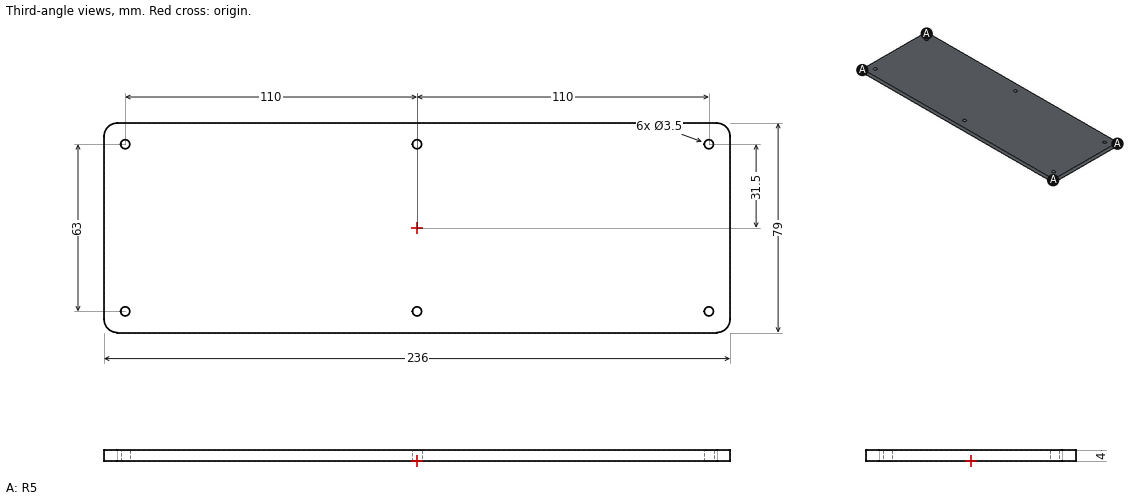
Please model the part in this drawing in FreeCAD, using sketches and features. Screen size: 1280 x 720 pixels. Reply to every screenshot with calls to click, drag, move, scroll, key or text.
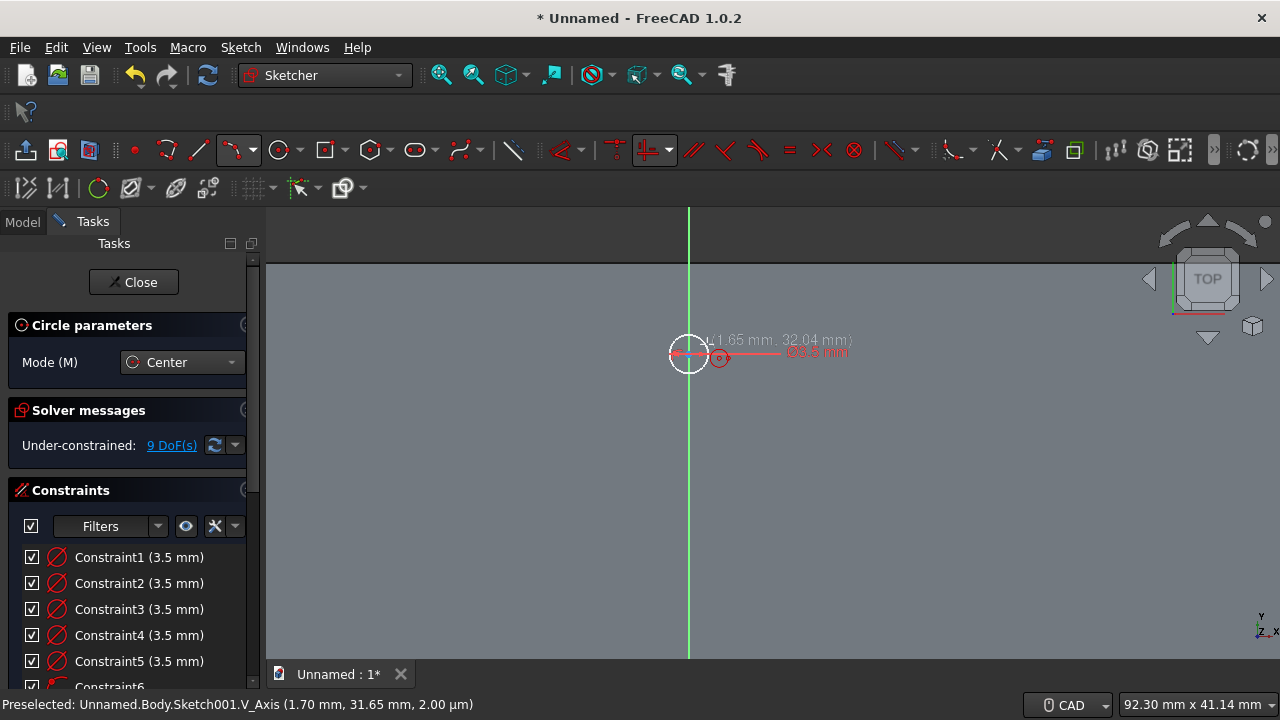
scroll(710, 347, down, 7)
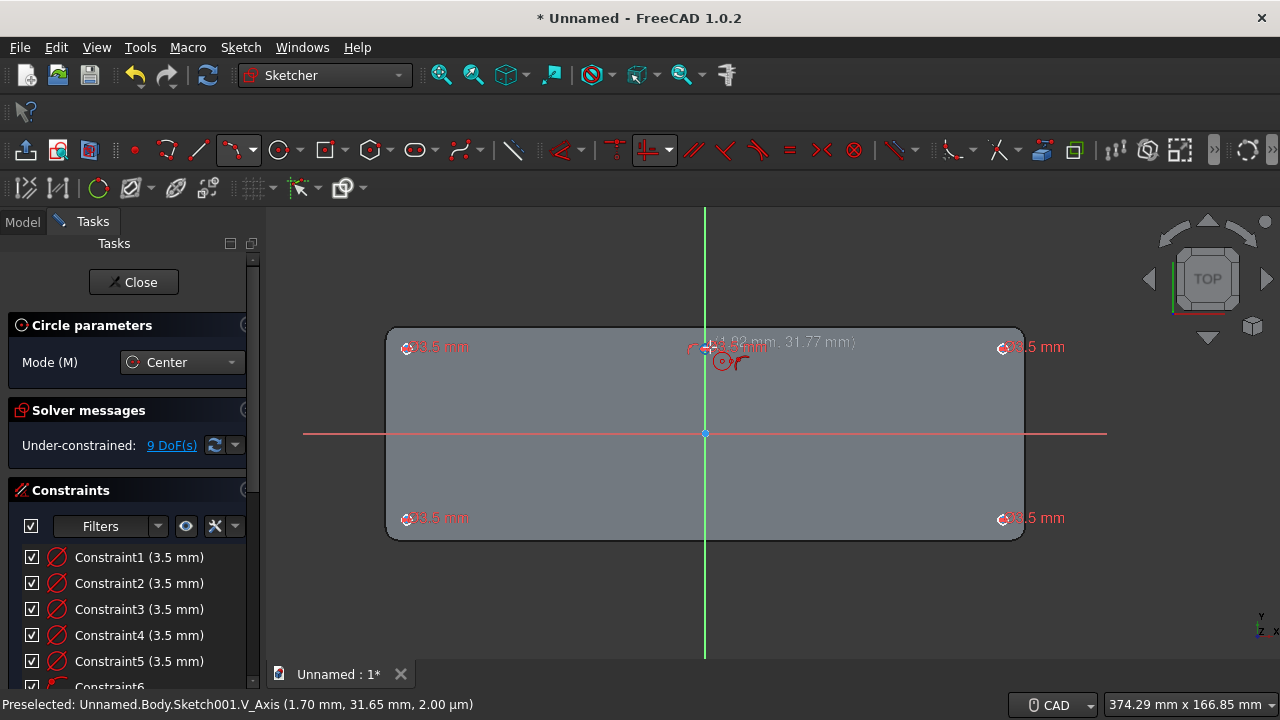
scroll(705, 519, up, 8)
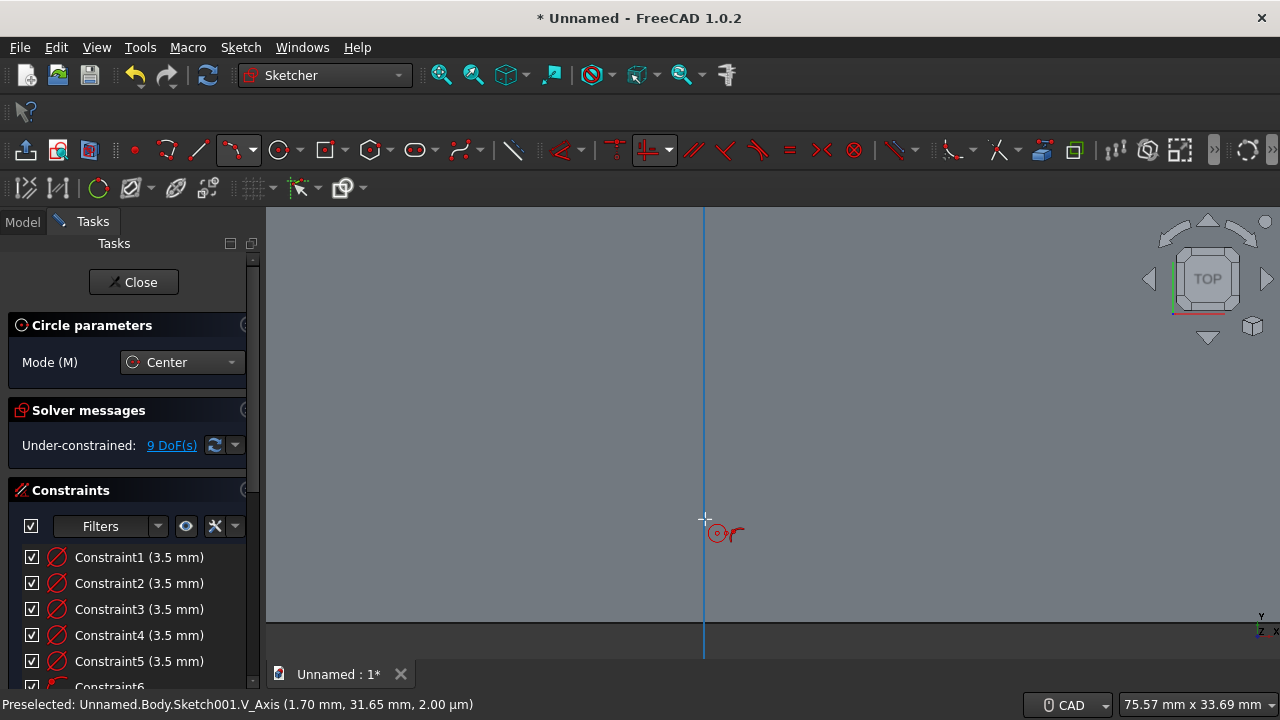
scroll(705, 519, down, 8)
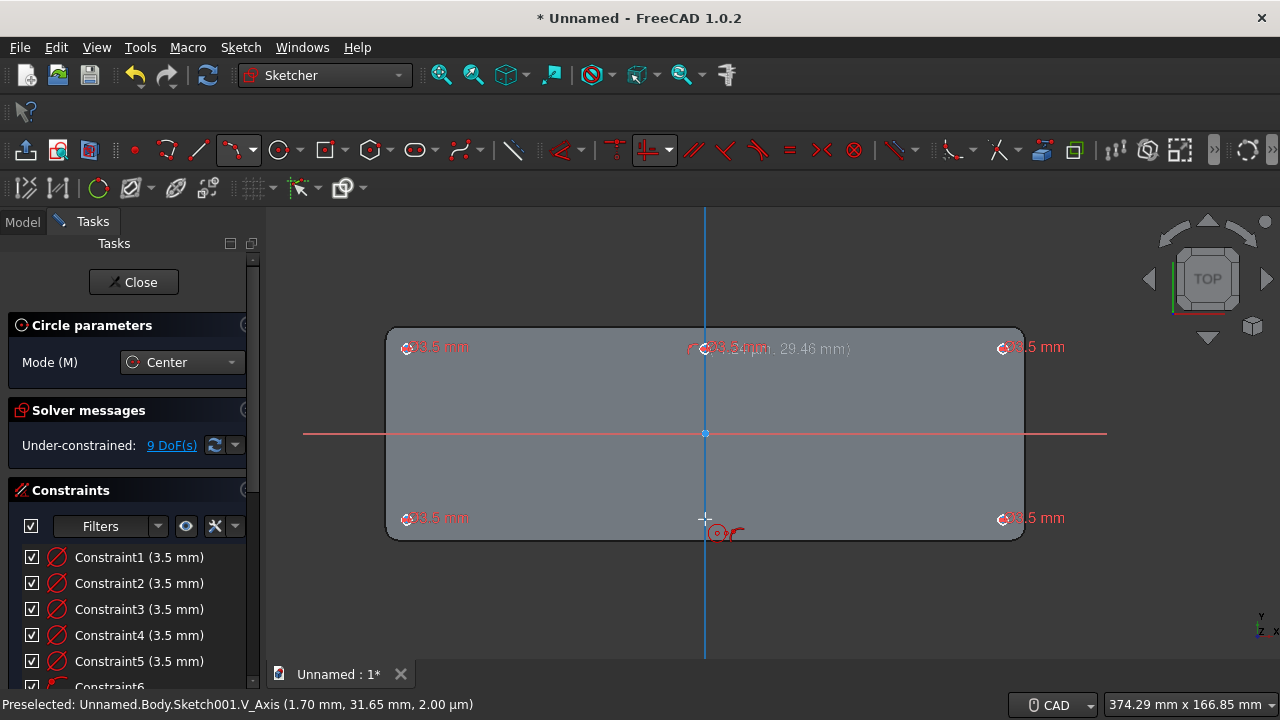
click(705, 519)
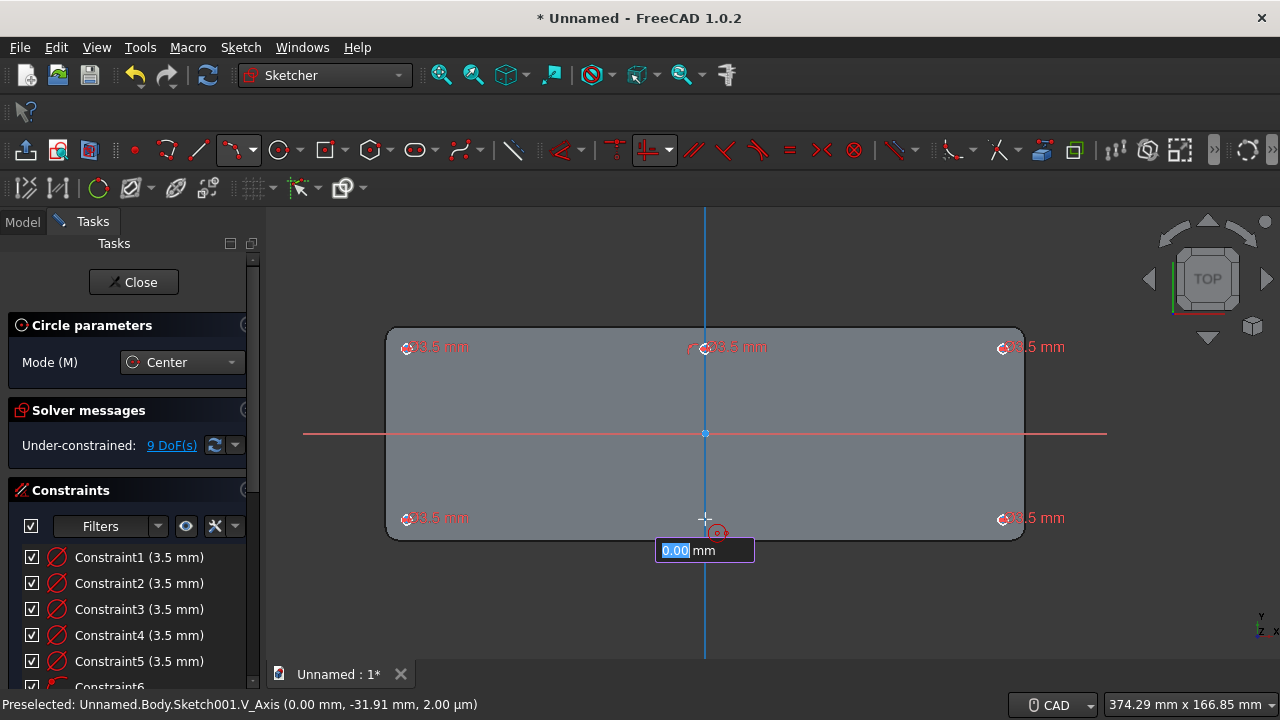
scroll(710, 517, up, 7)
move(707, 516)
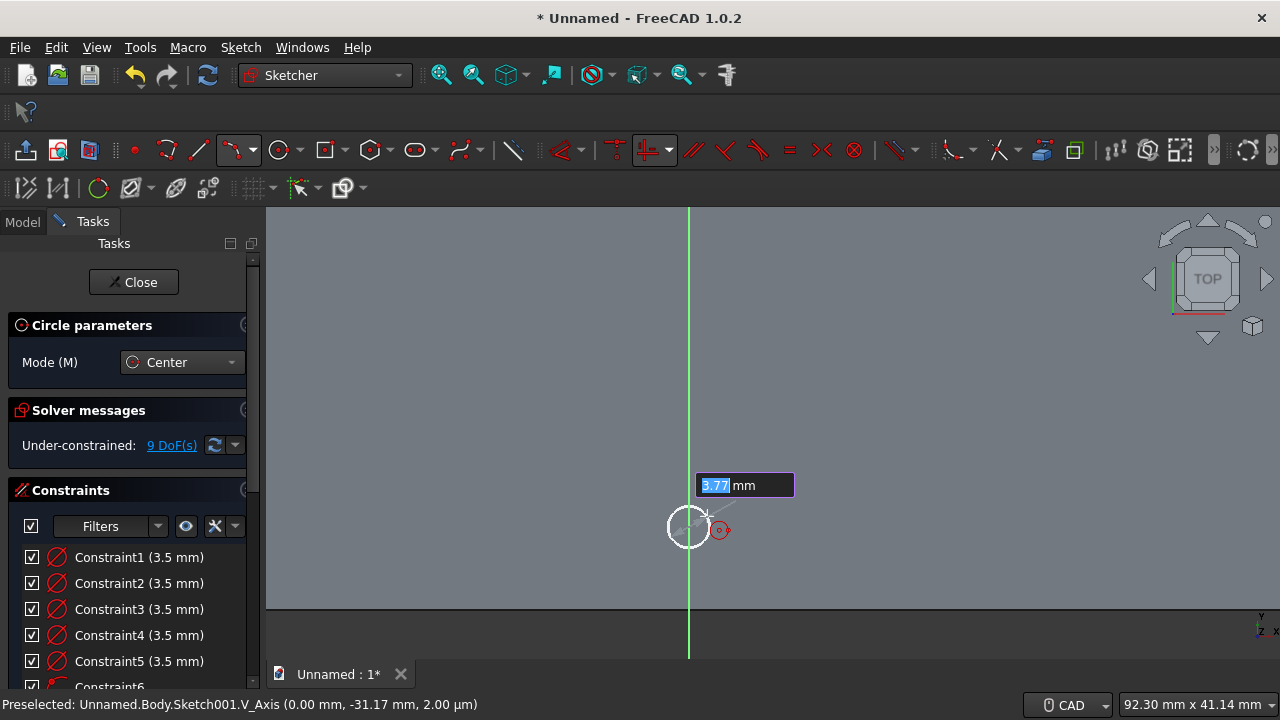
text(3.5)
key(Return)
key(Escape)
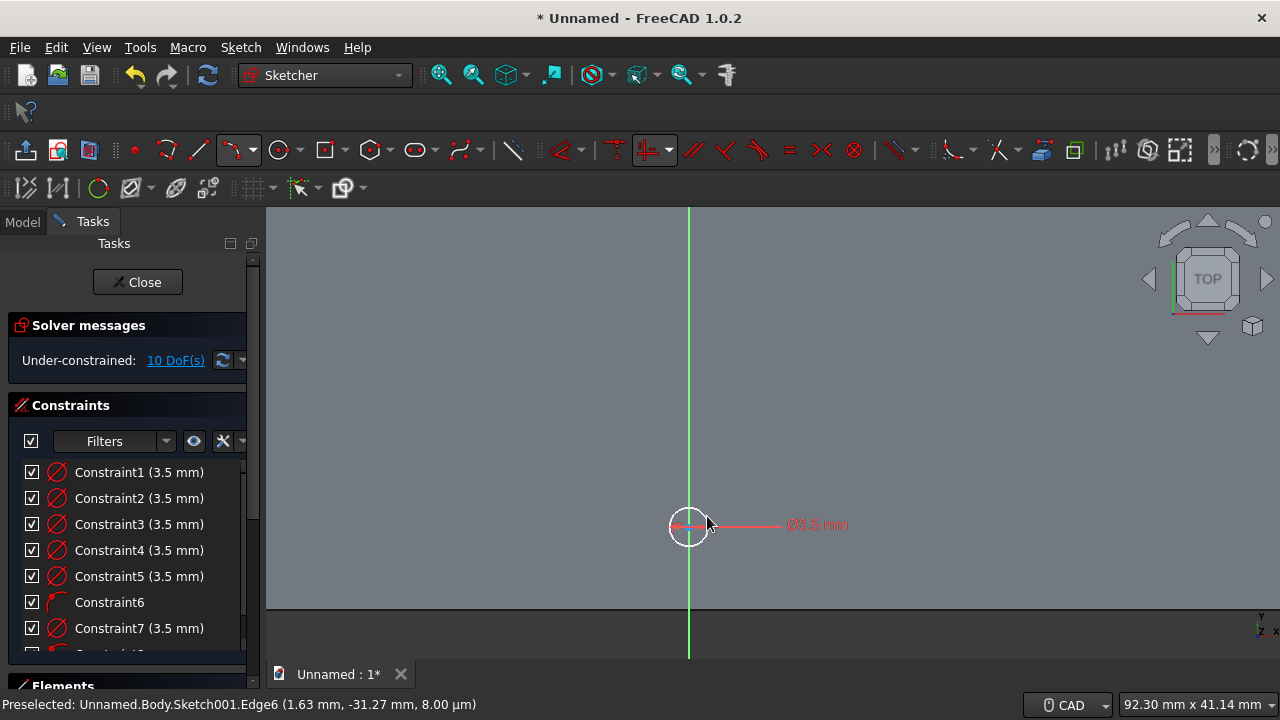
click(560, 150)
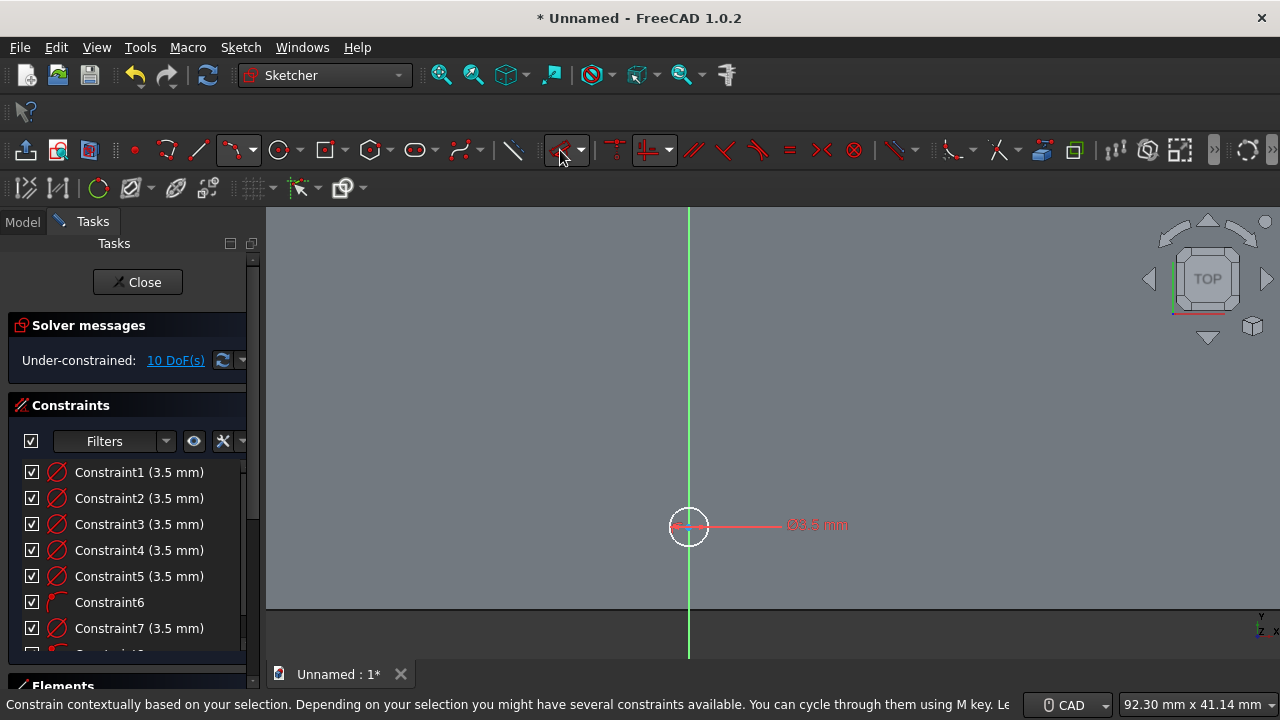
scroll(710, 517, down, 7)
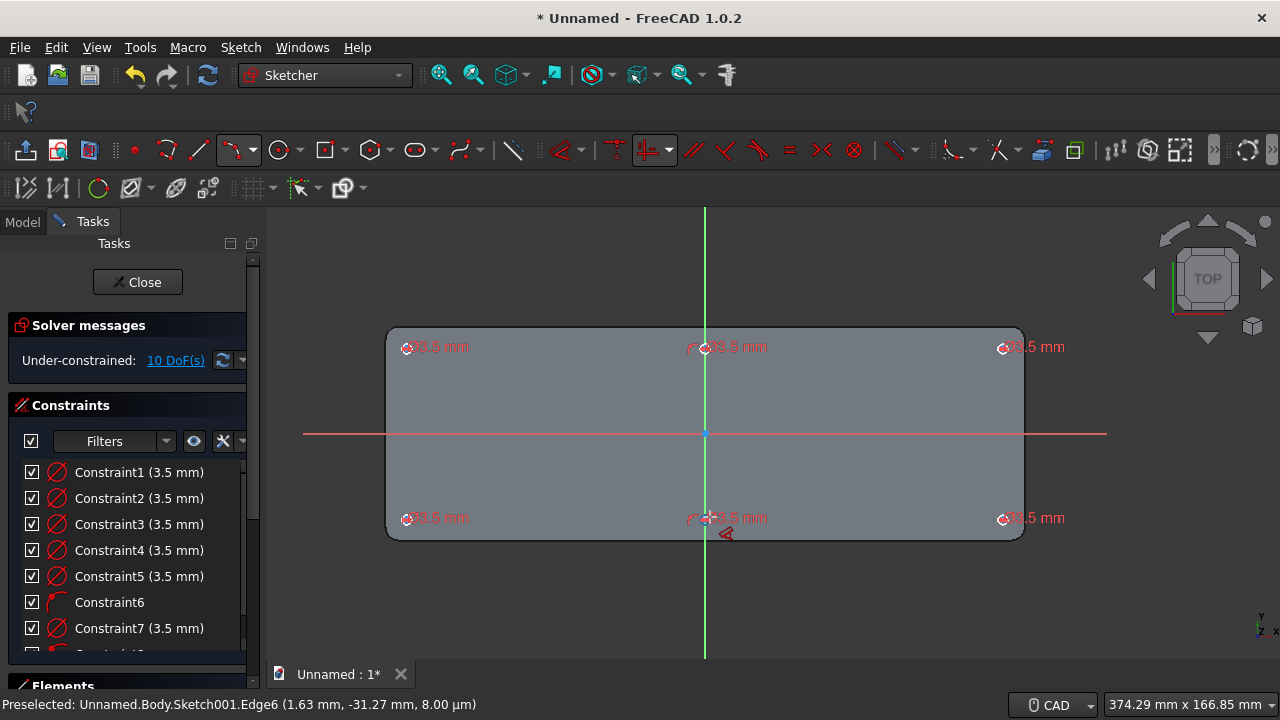
click(1003, 349)
click(854, 315)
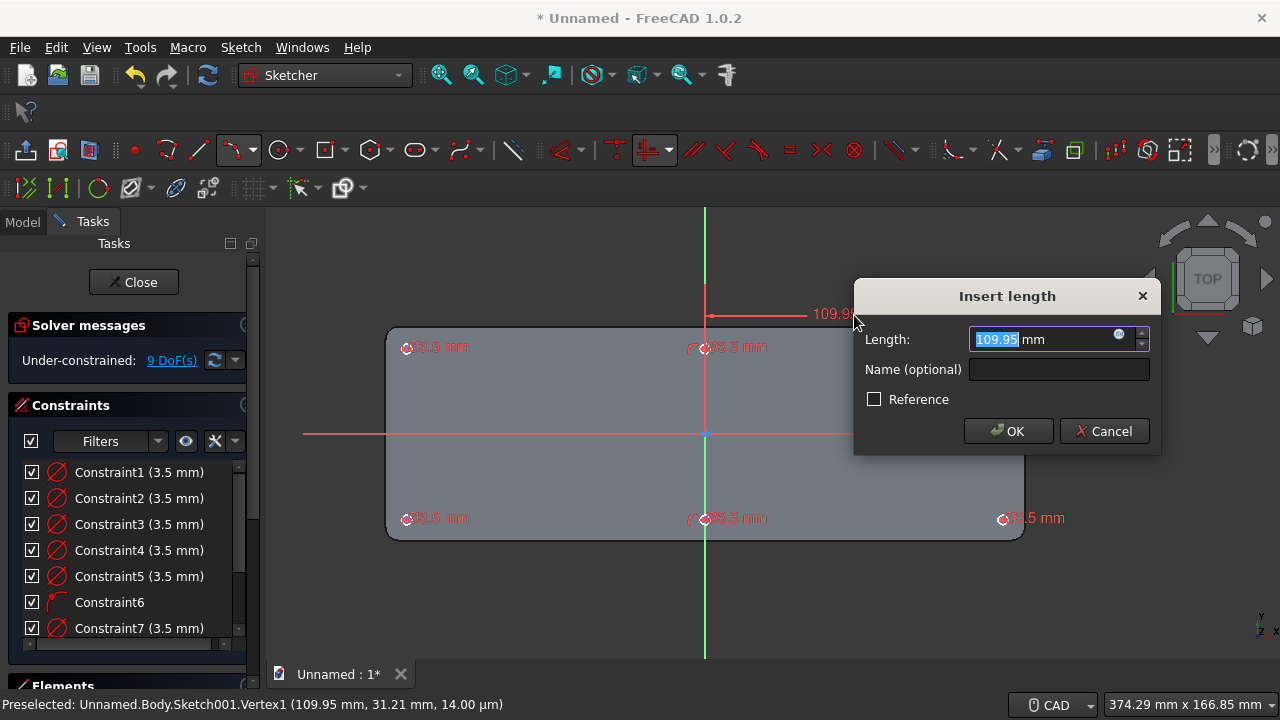
text(110)
key(Return)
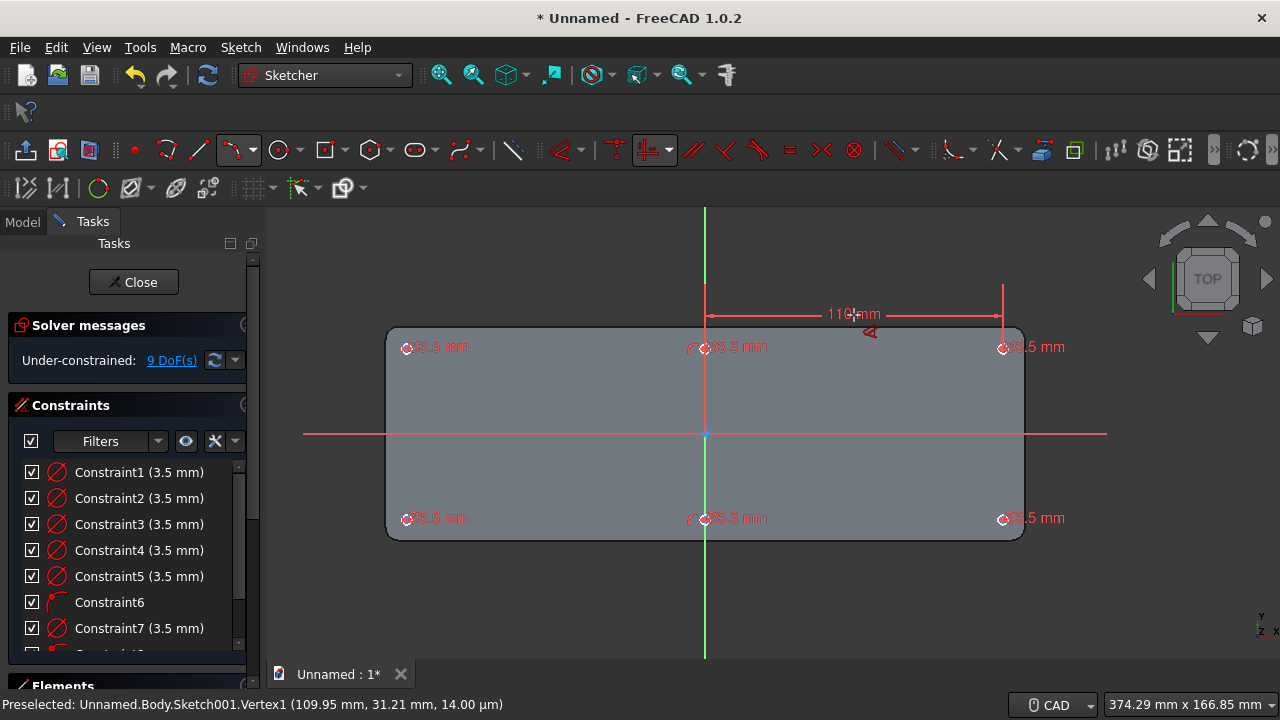
click(407, 349)
click(556, 315)